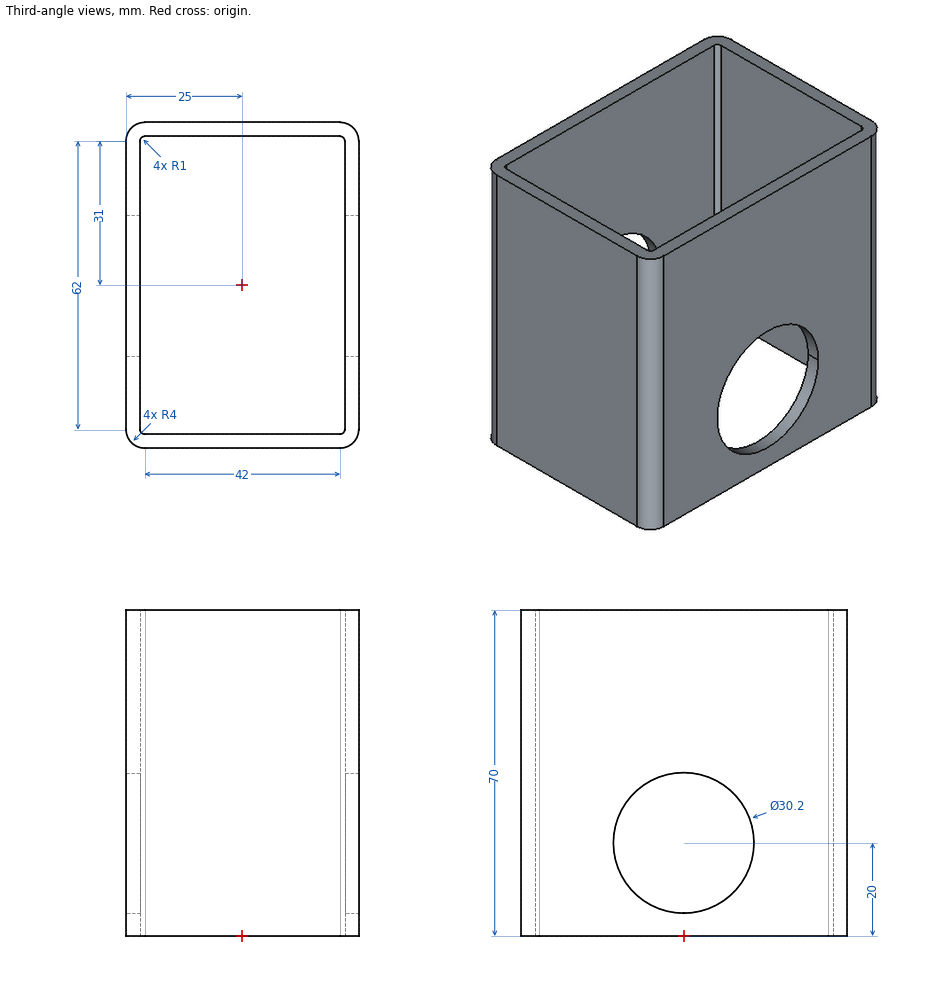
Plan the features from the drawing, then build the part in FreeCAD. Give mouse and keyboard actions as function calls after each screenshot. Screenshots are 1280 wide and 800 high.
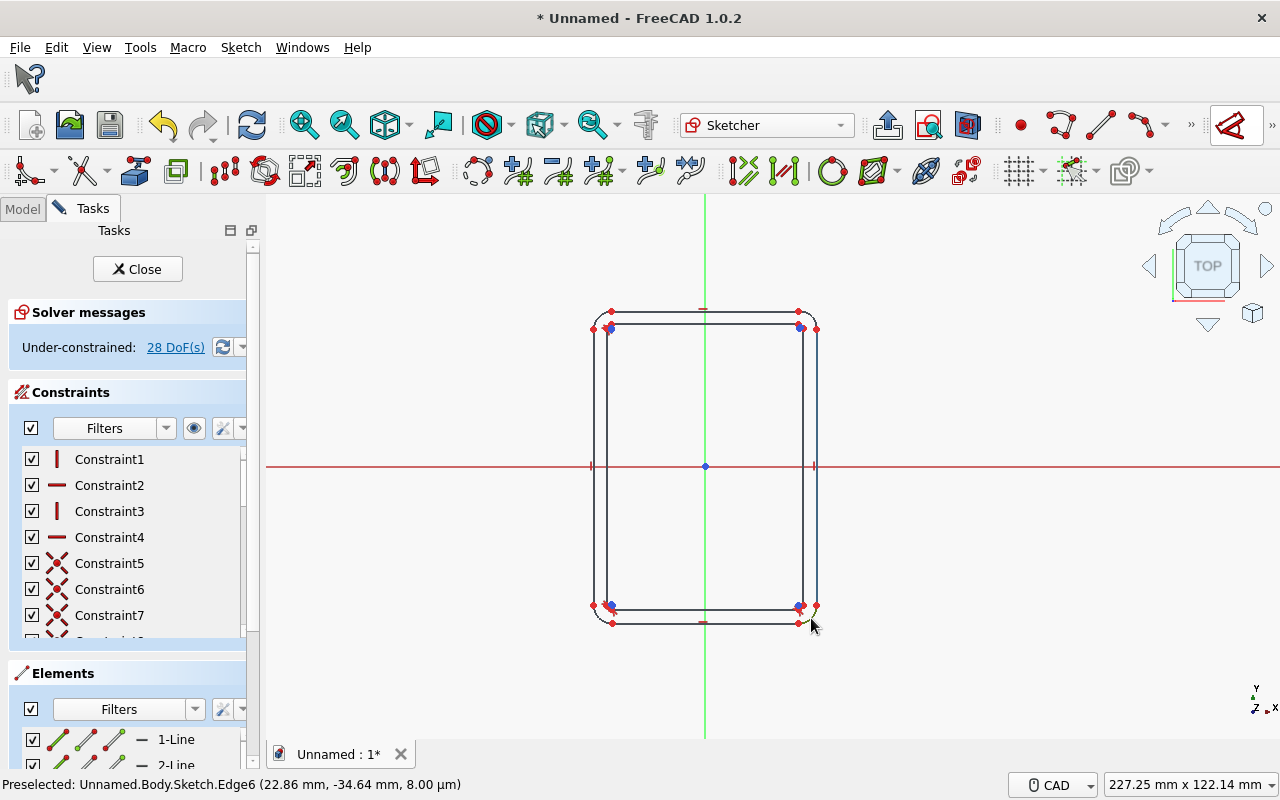
key(t)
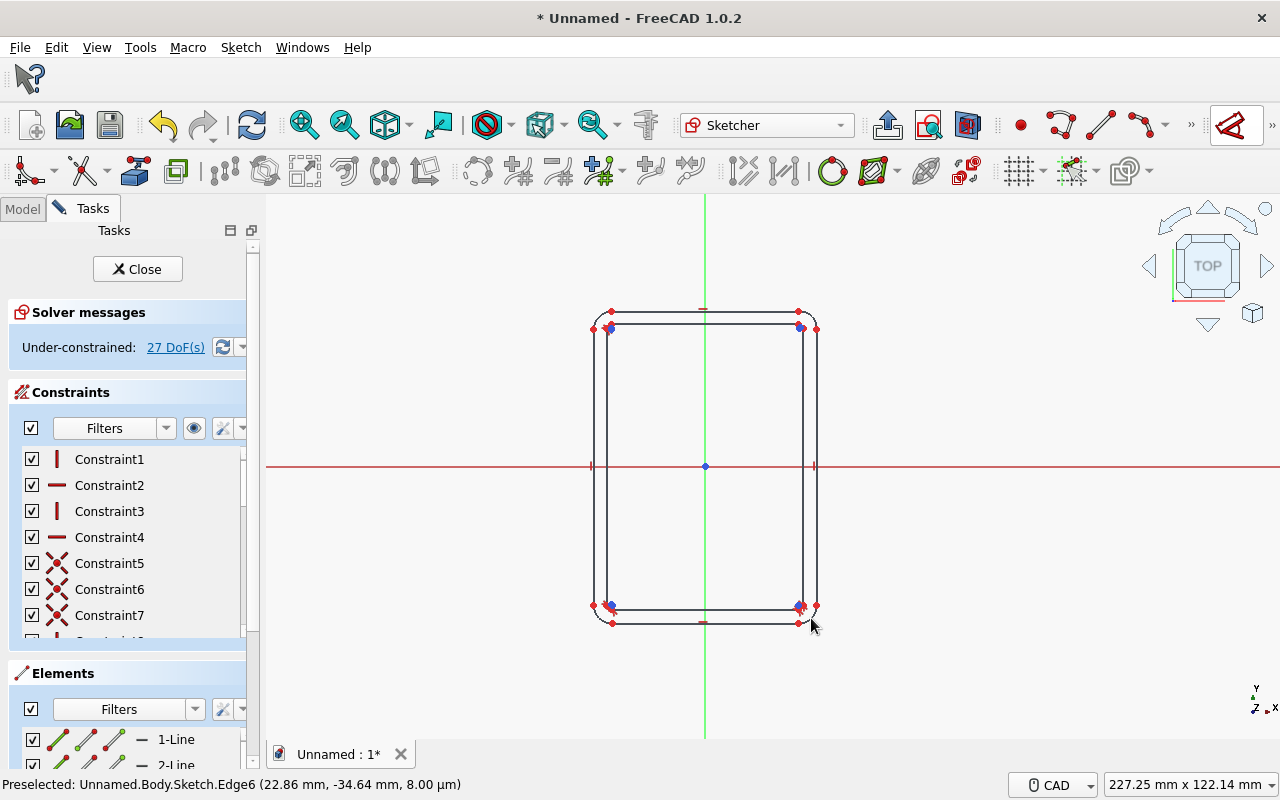
click(817, 523)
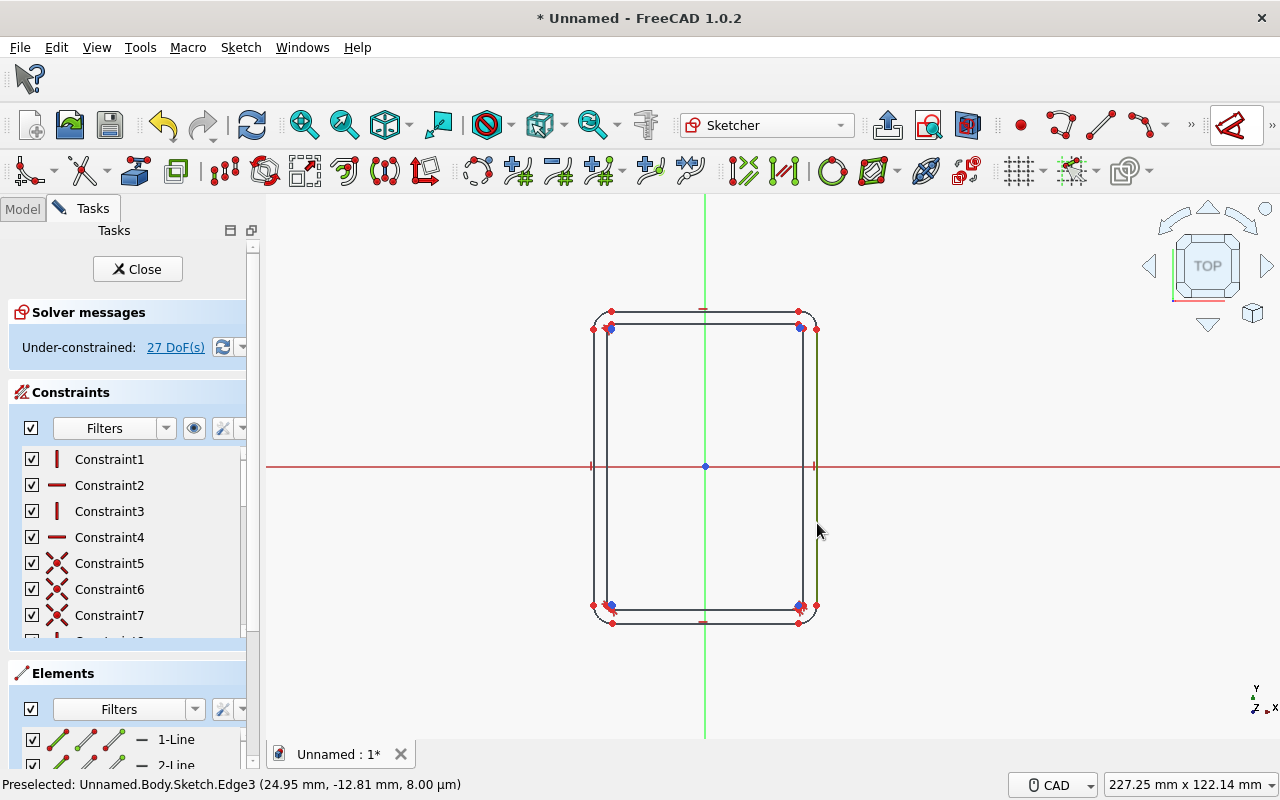
click(812, 316)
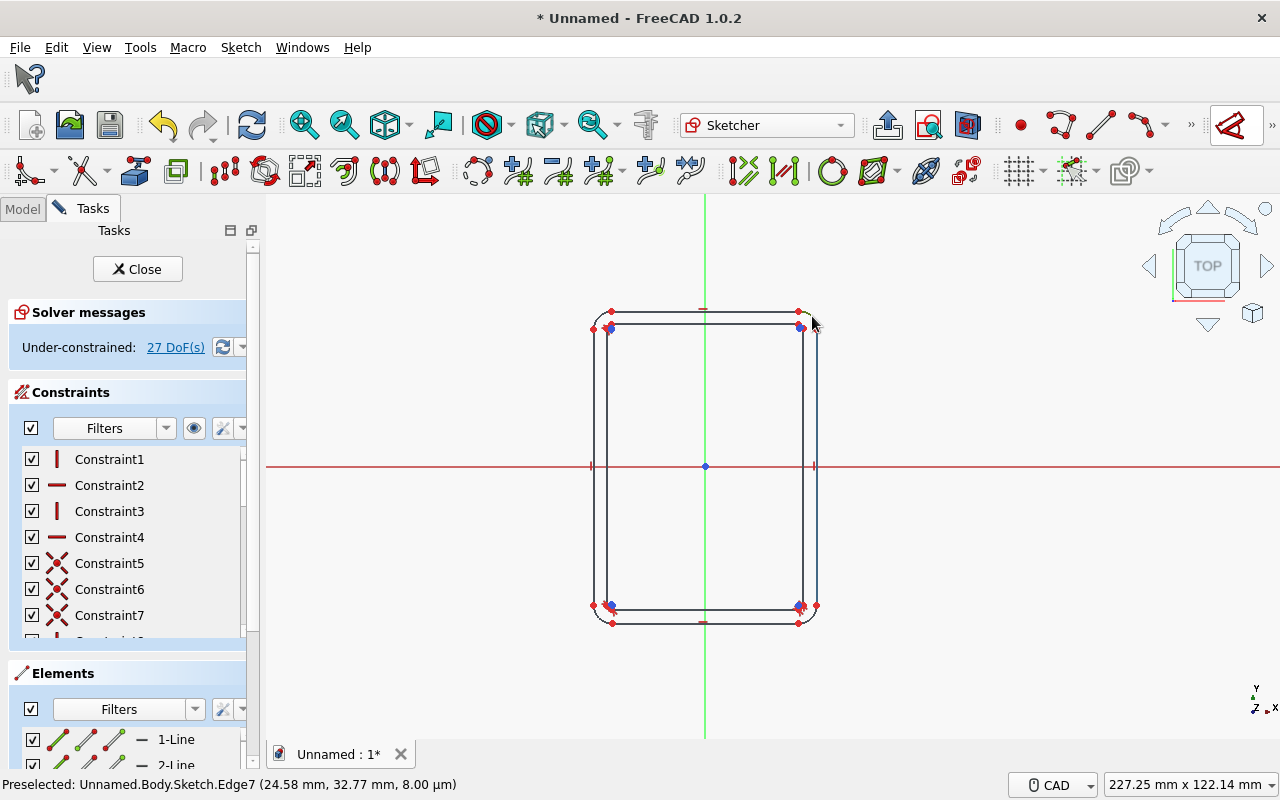
key(t)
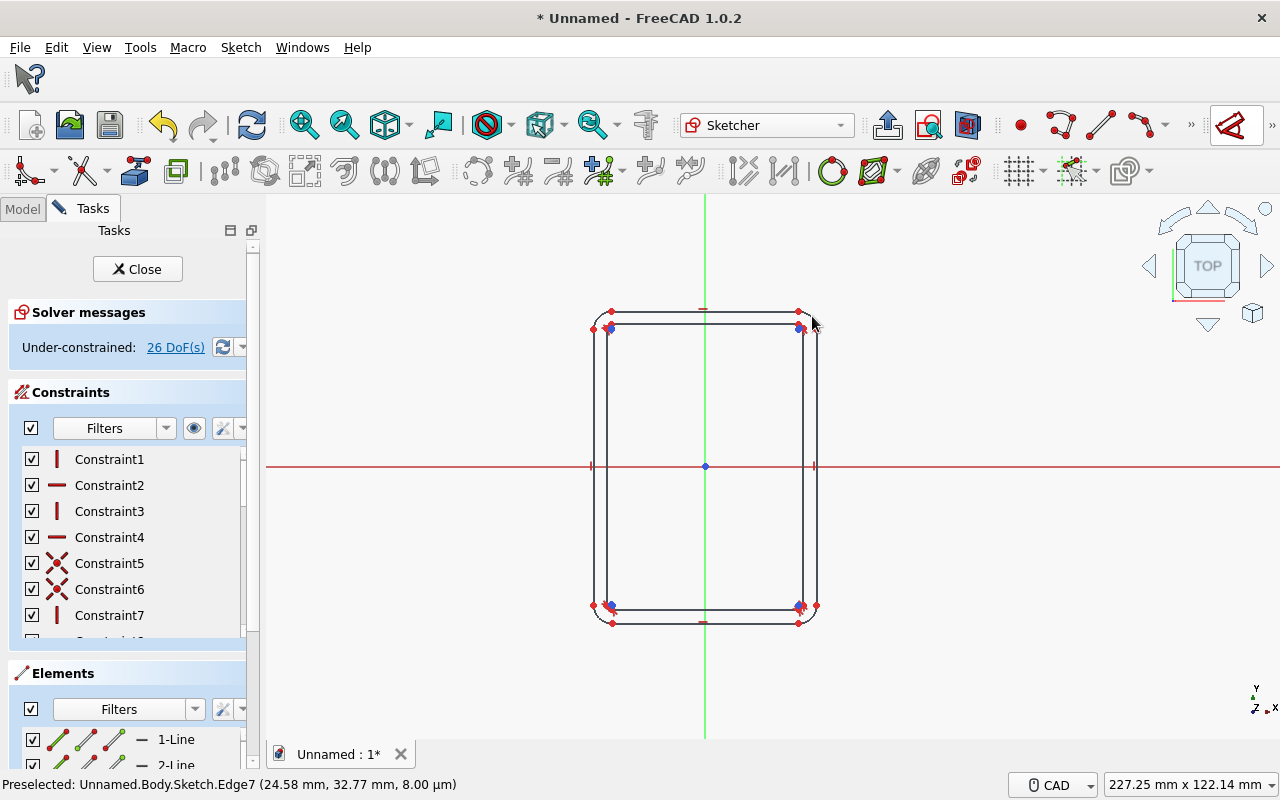
click(743, 312)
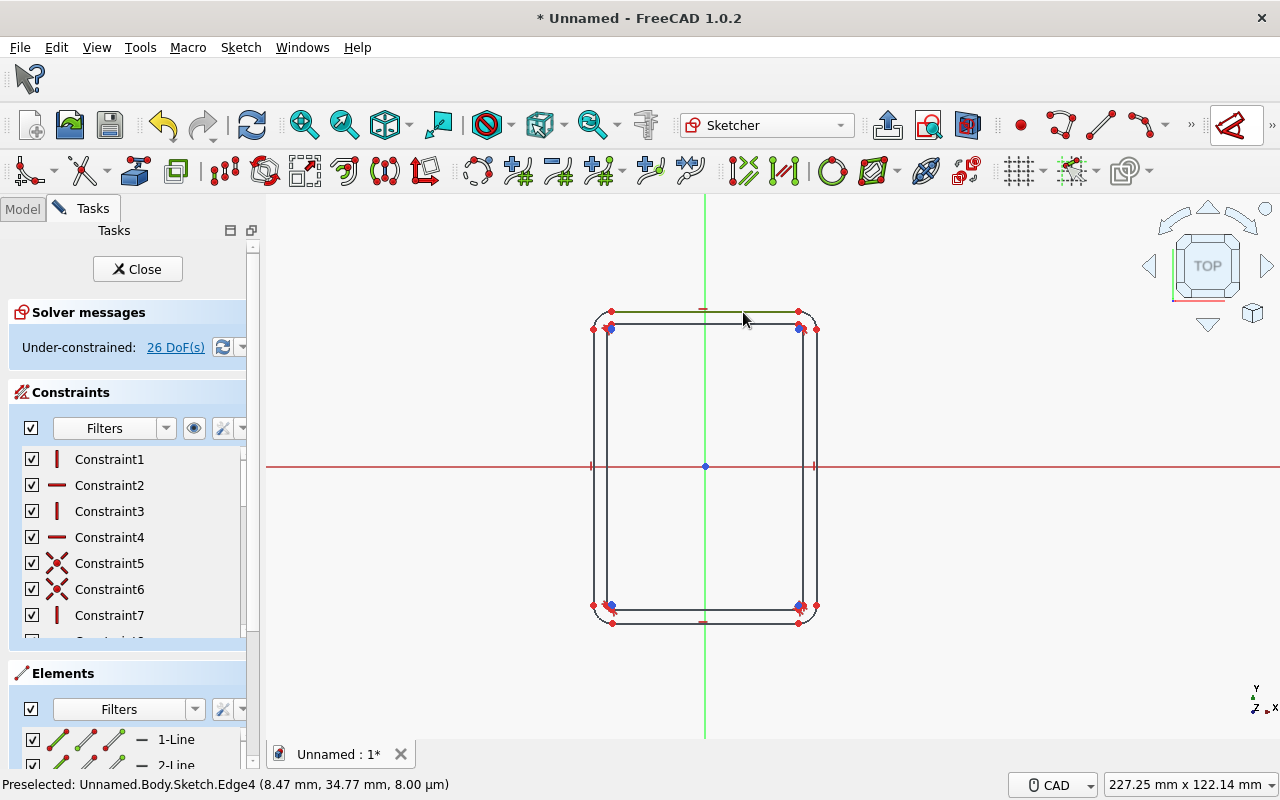
click(811, 317)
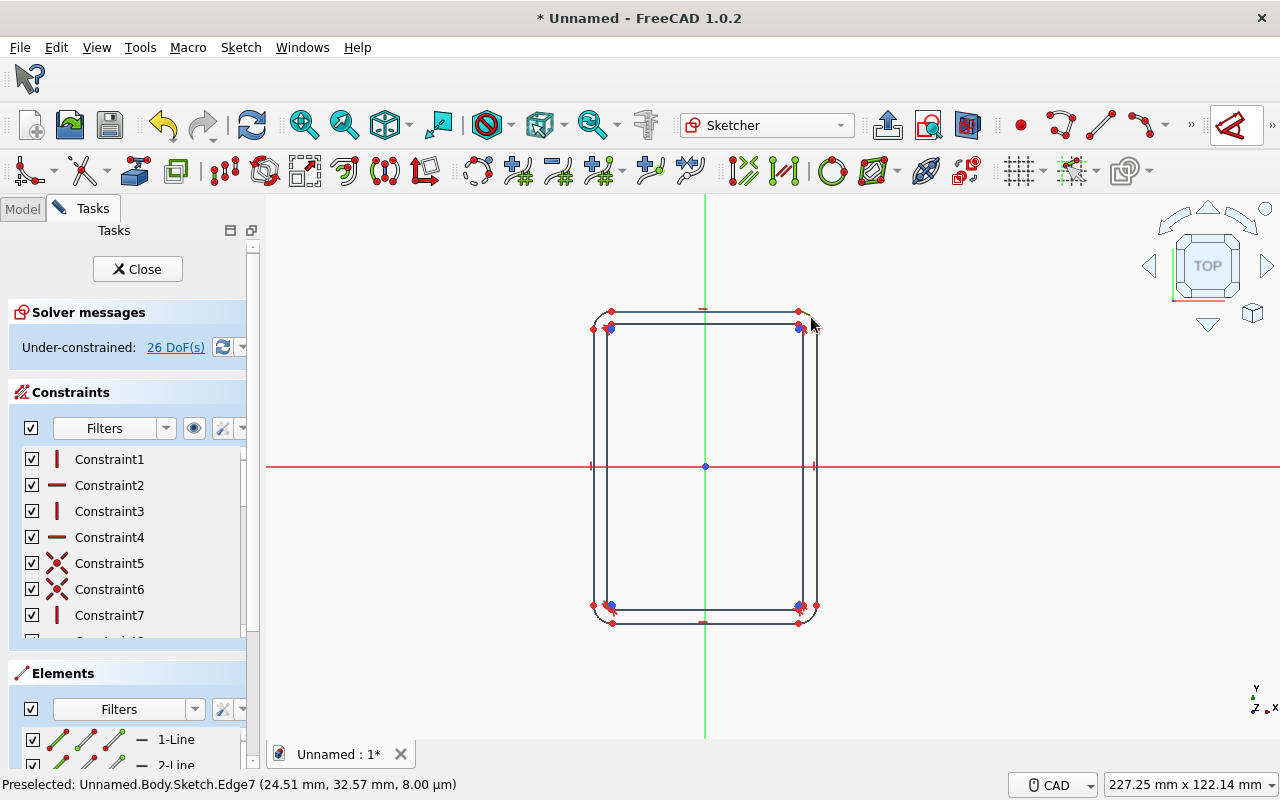
key(t)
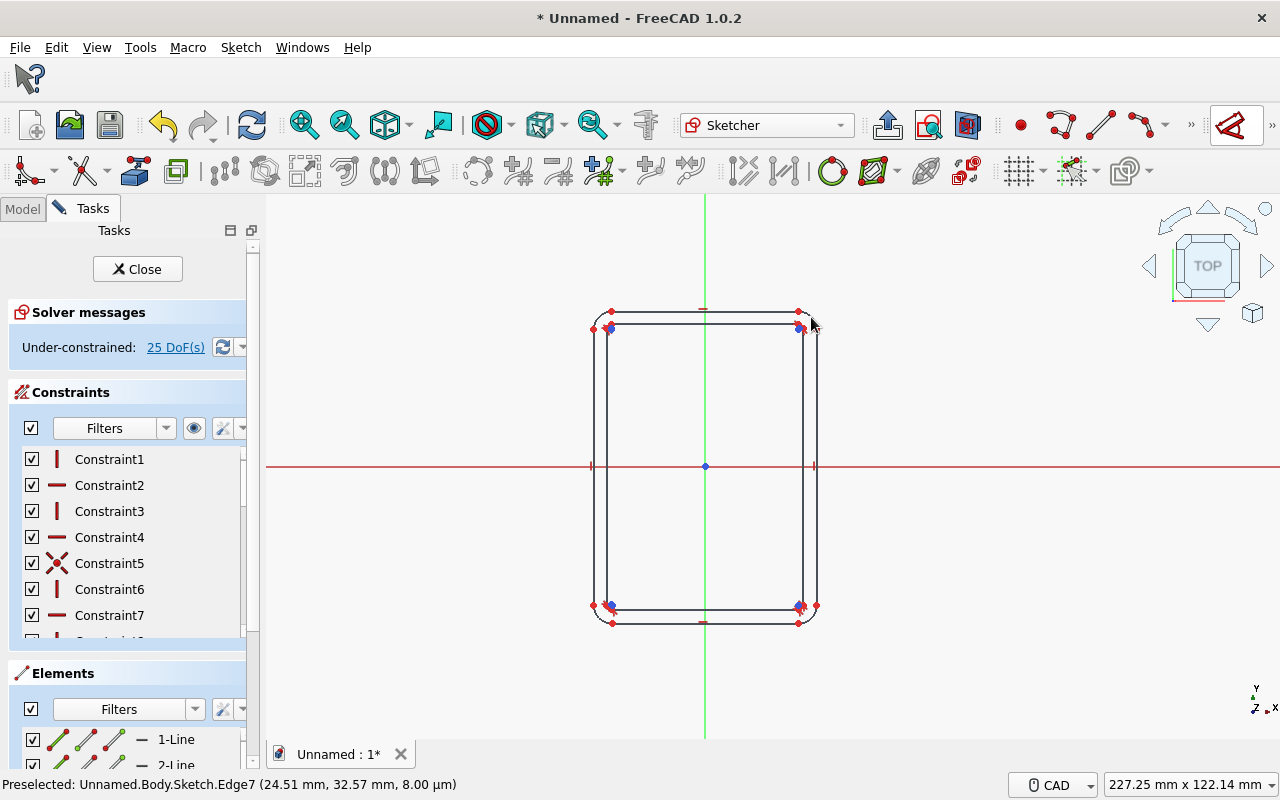
click(743, 312)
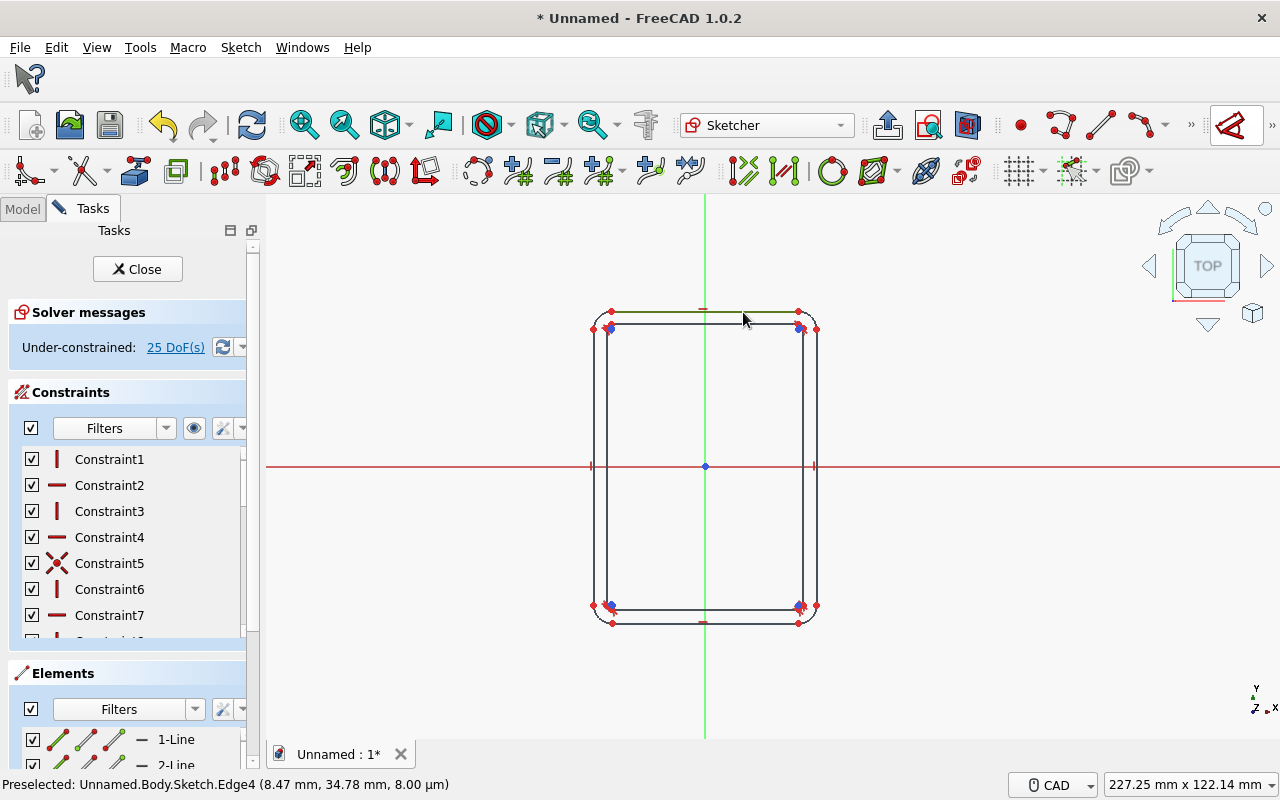
click(599, 317)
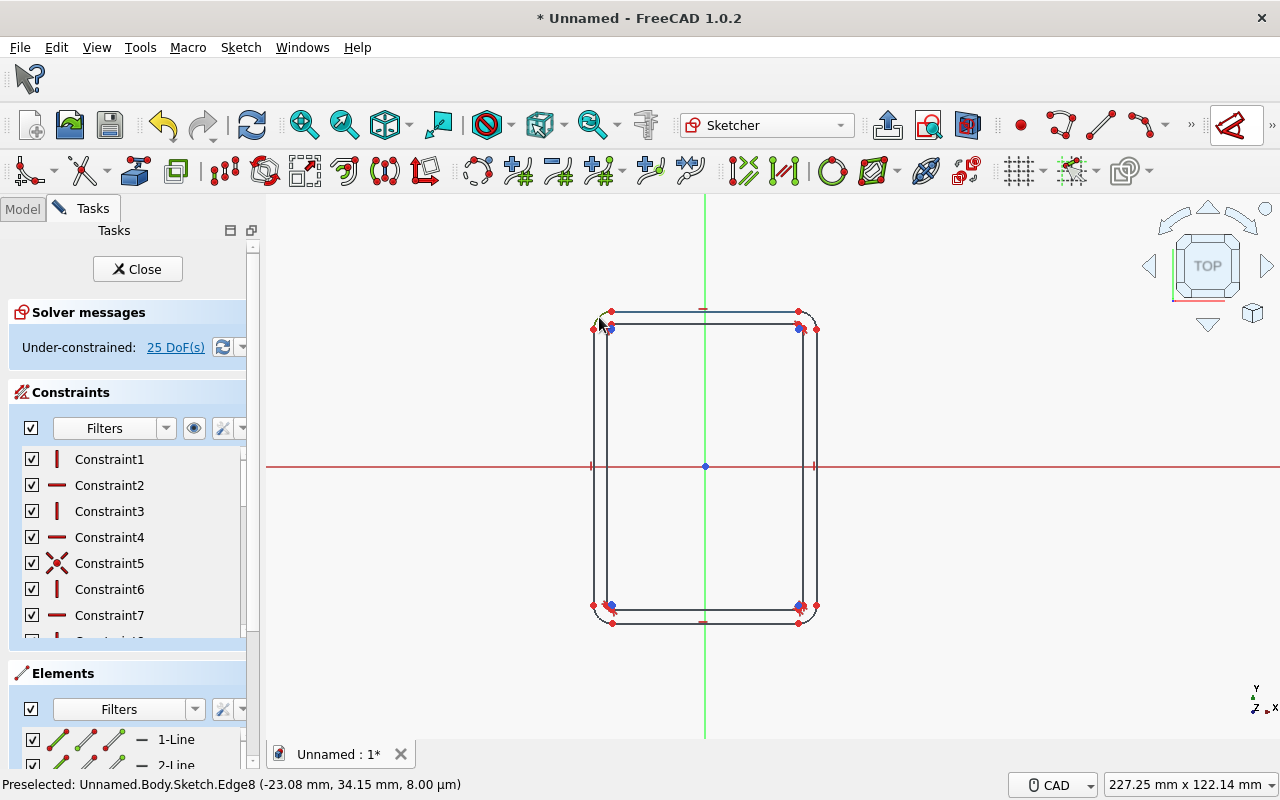
key(t)